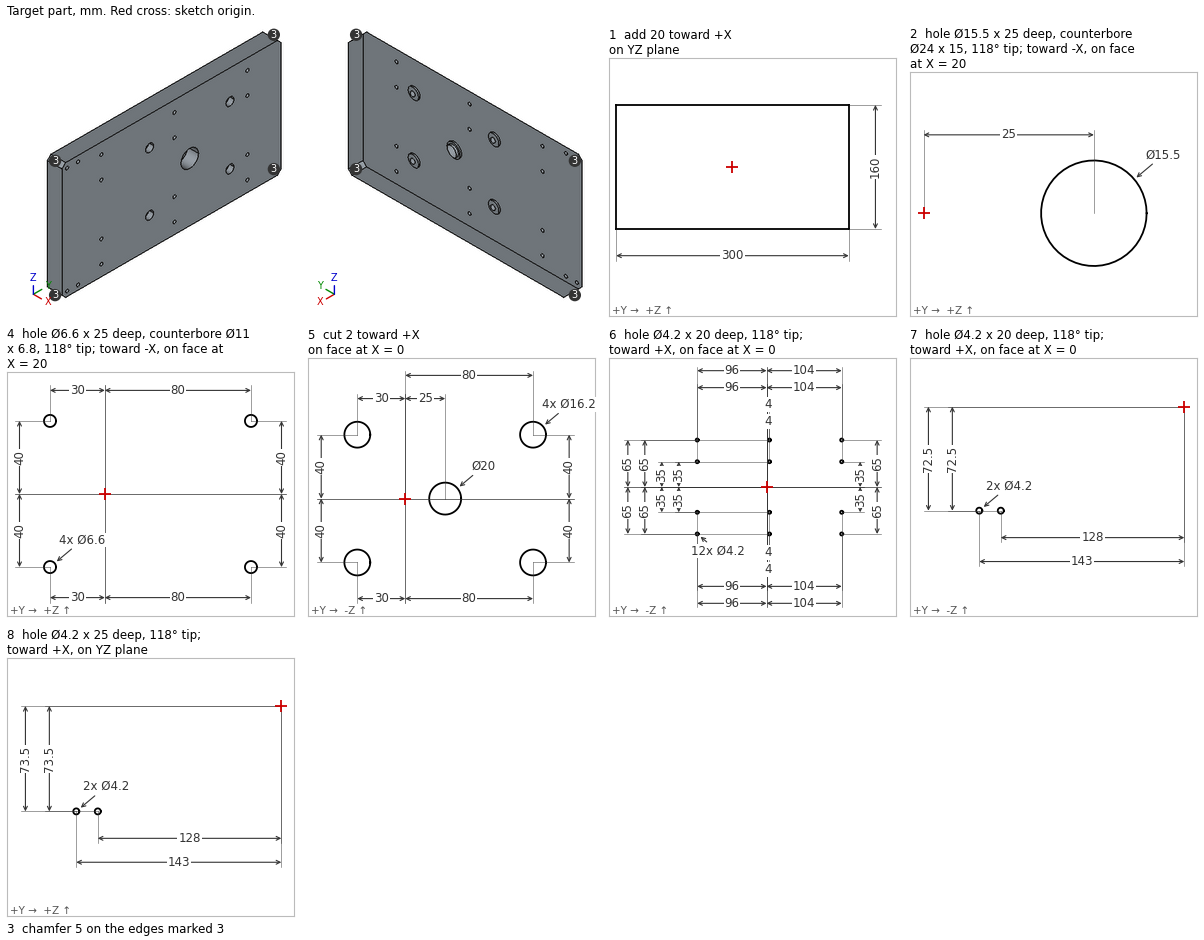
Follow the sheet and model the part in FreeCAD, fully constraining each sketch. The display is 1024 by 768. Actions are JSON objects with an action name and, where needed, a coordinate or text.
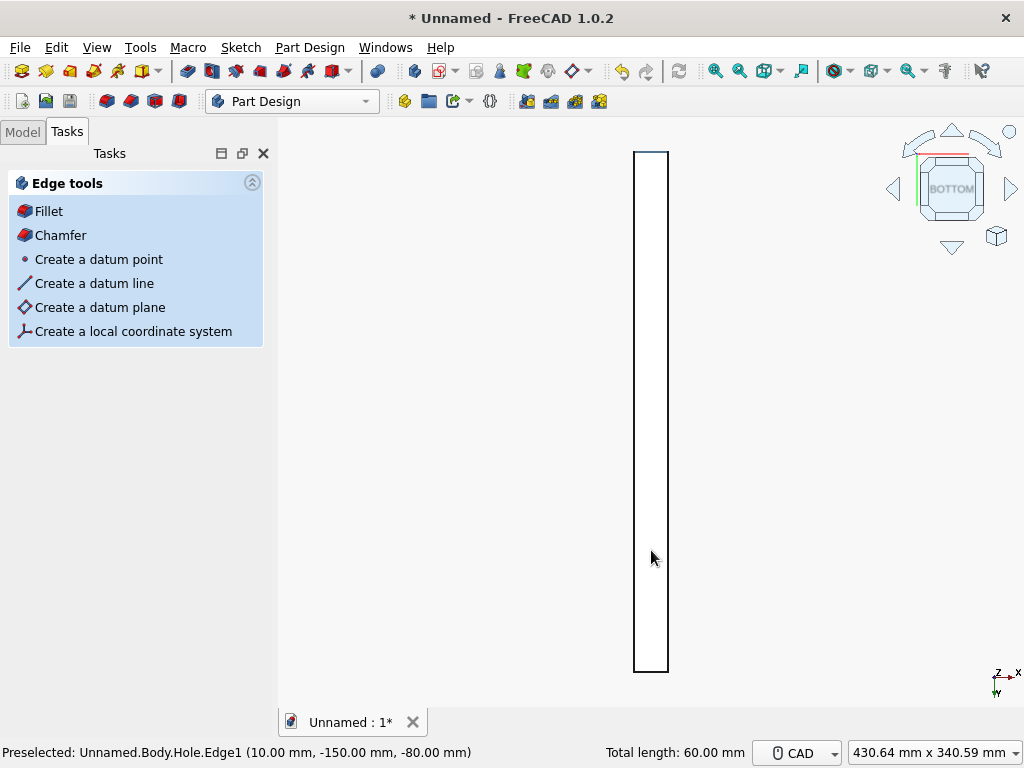
{"action": "left_click", "coordinate": [651, 671], "text": "ctrl"}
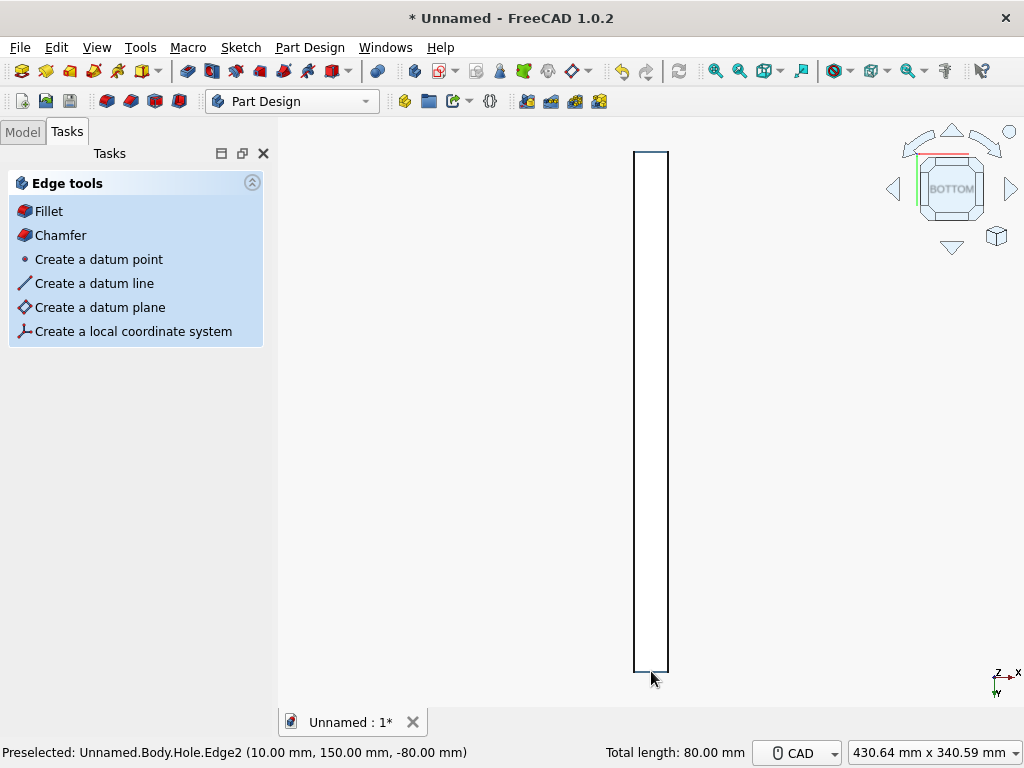
{"action": "left_click", "coordinate": [132, 102]}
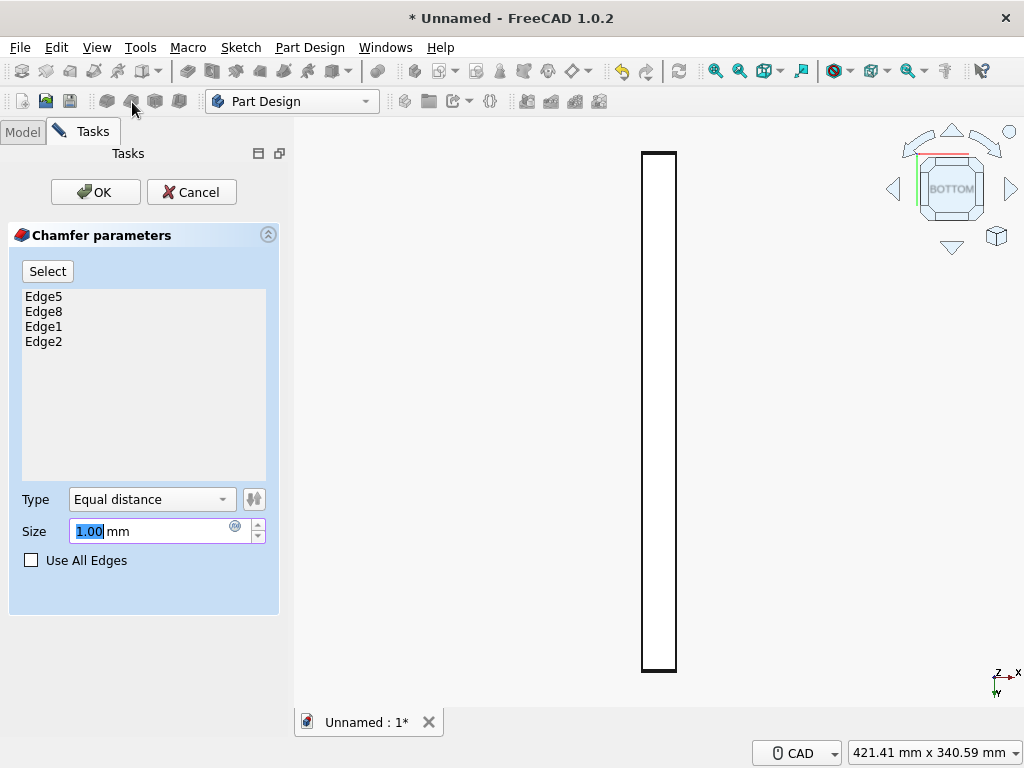
{"action": "type", "text": "5"}
{"action": "key", "text": "Tab"}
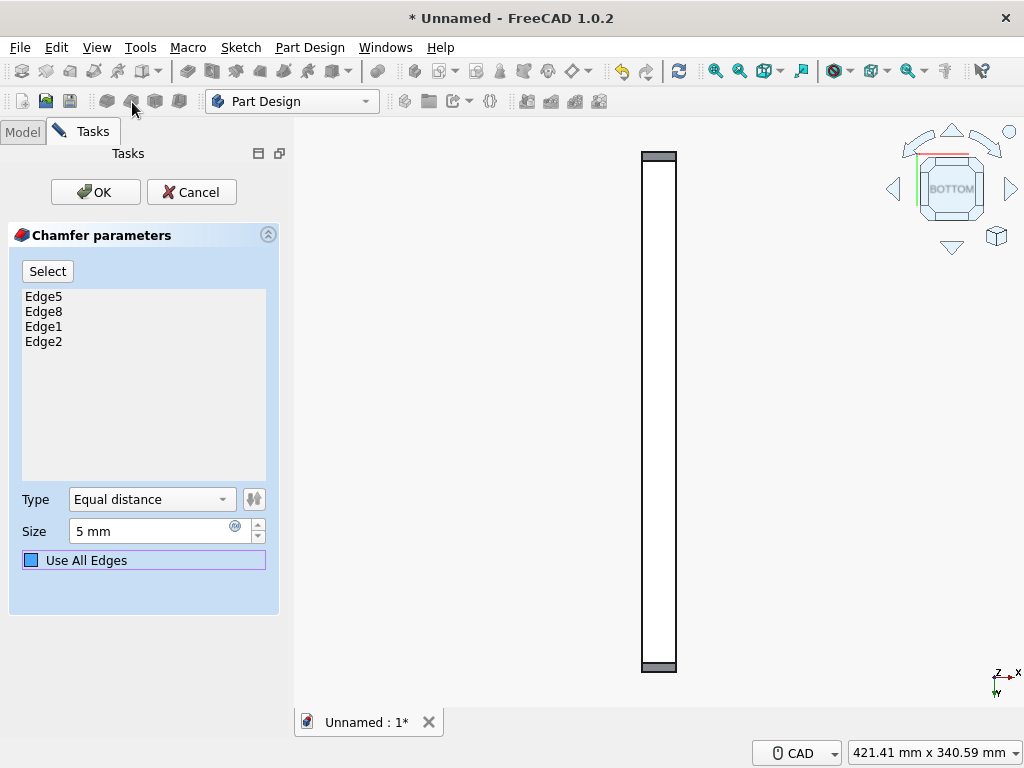
{"action": "left_click", "coordinate": [96, 192]}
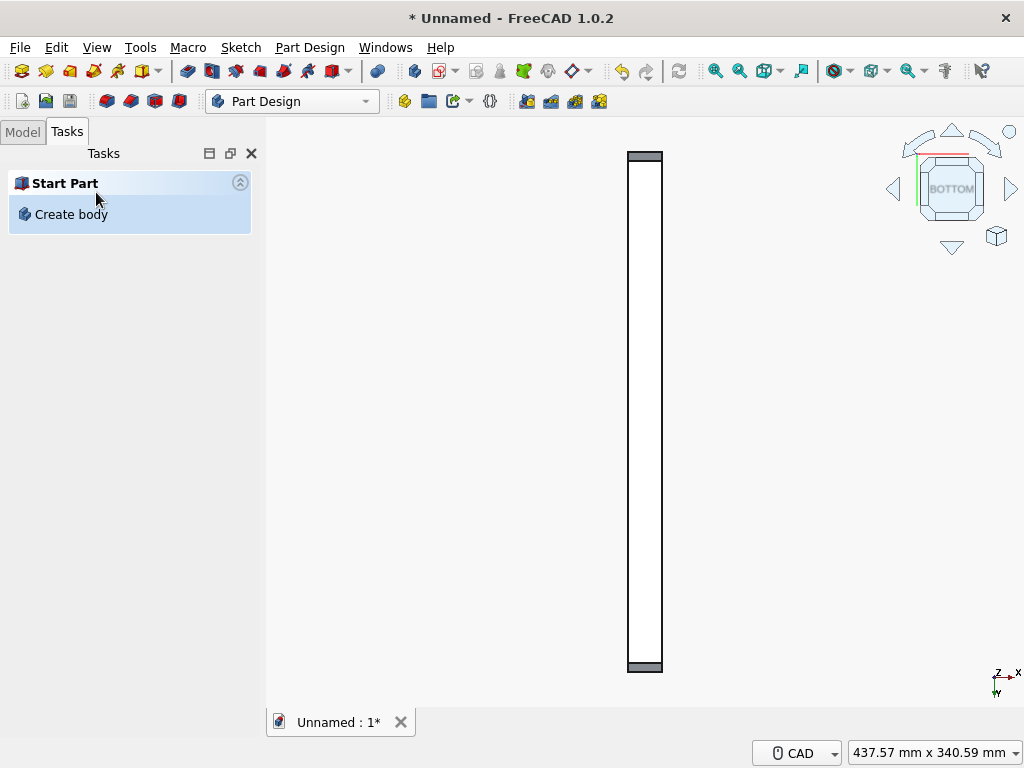
{"action": "key", "text": "0"}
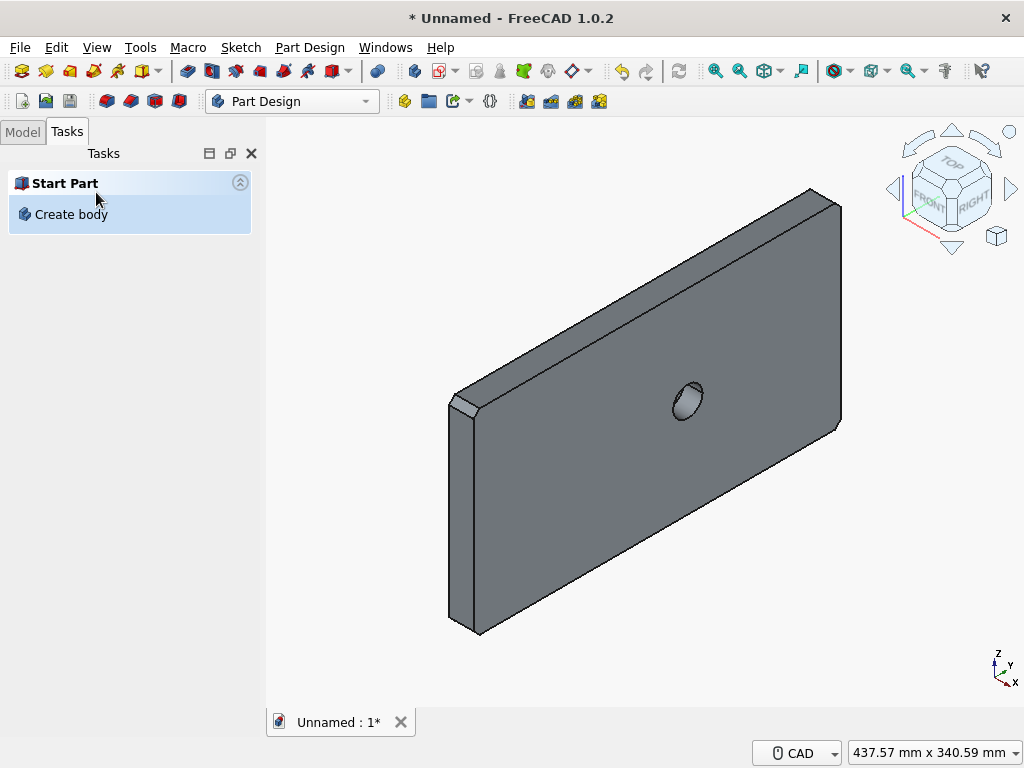
{"action": "left_click", "coordinate": [552, 479]}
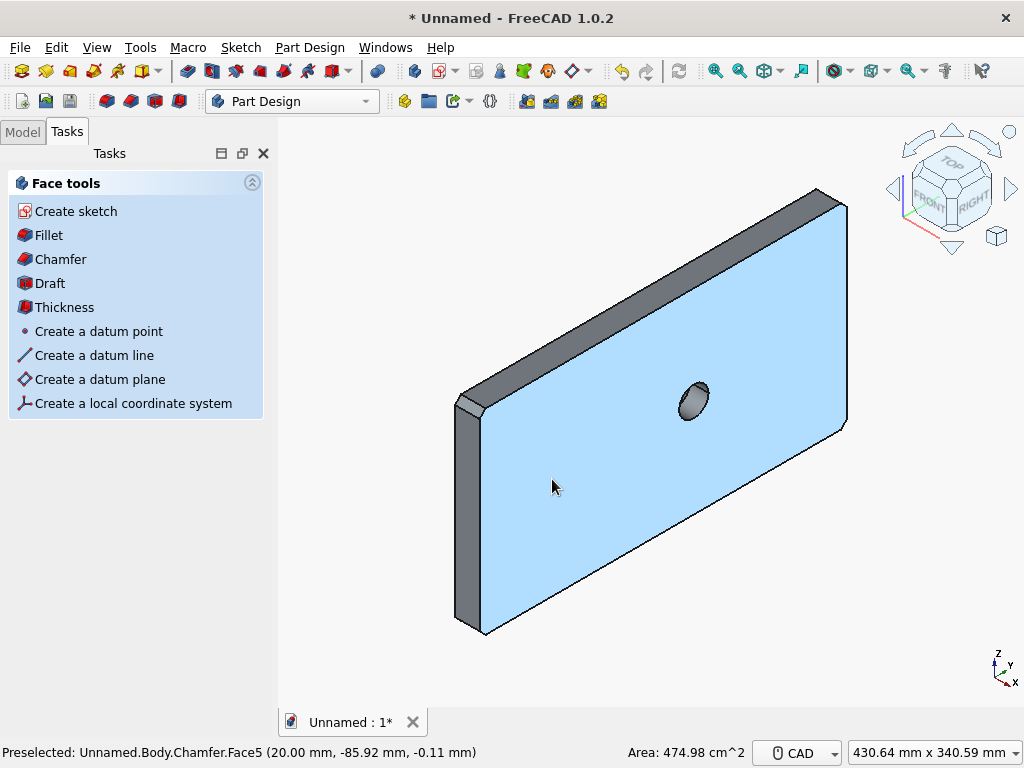
{"action": "left_click", "coordinate": [440, 72]}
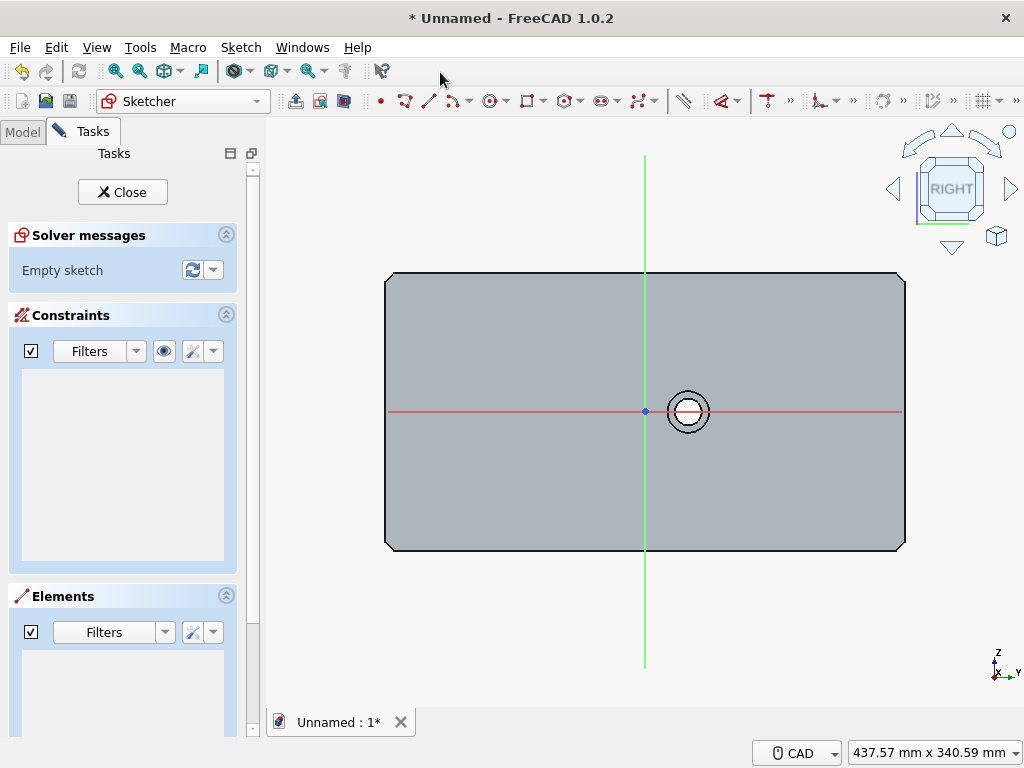
{"action": "scroll", "coordinate": [824, 412], "scroll_direction": "up", "scroll_amount": 3}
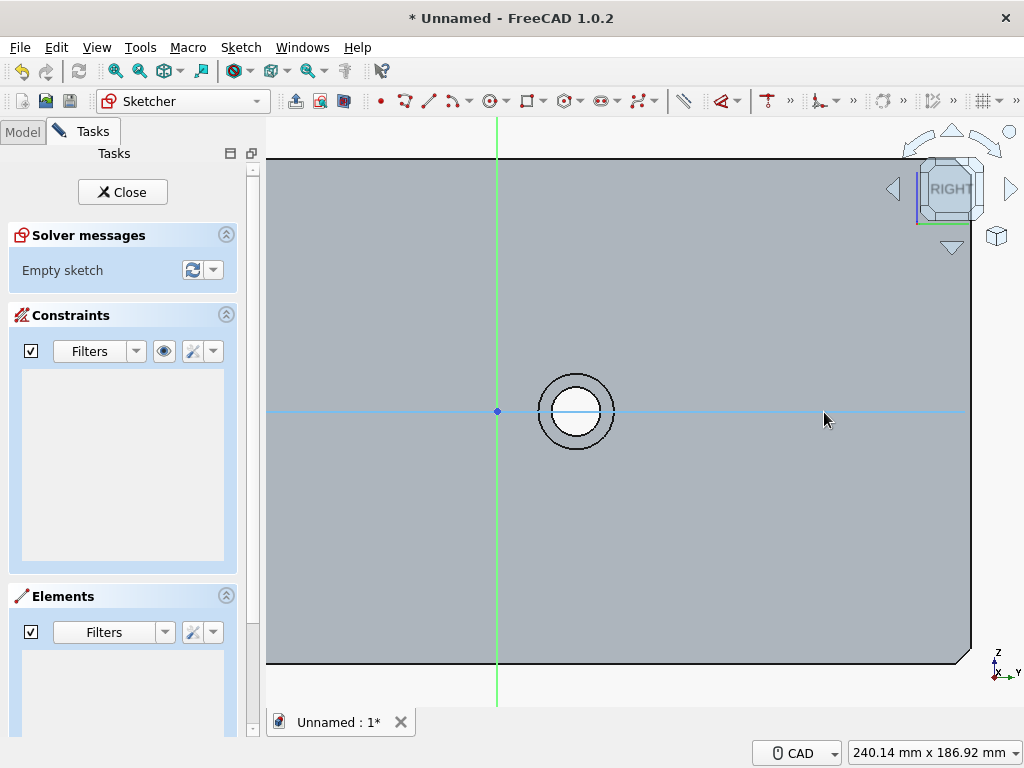
{"action": "left_click", "coordinate": [490, 102]}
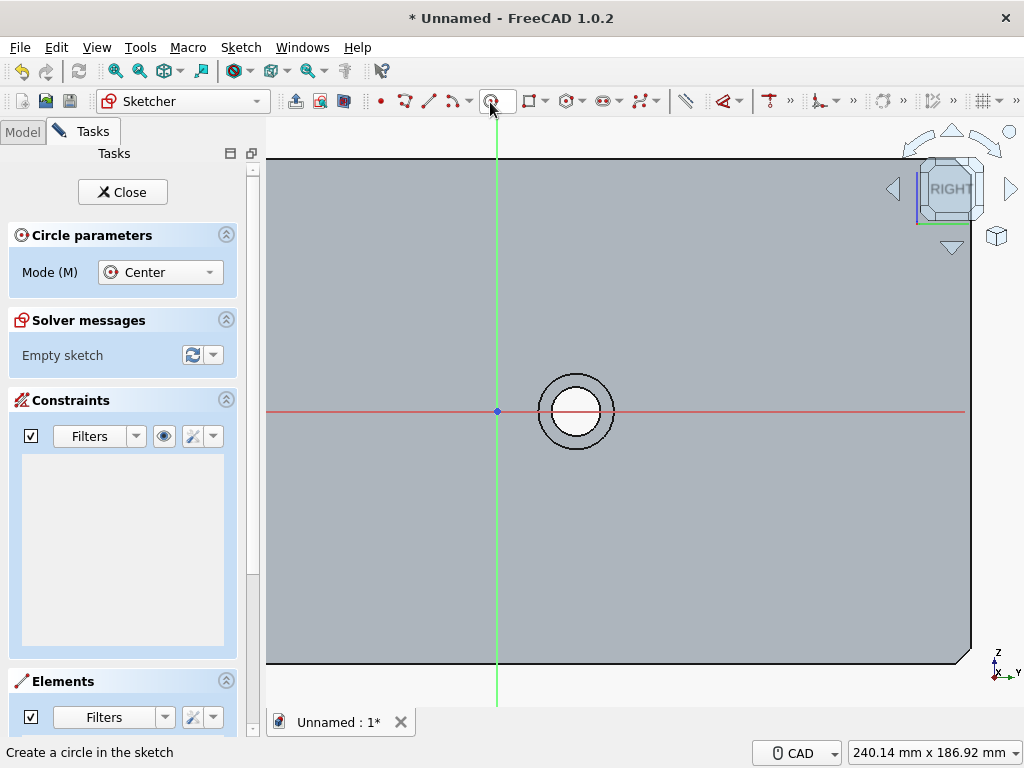
{"action": "scroll", "coordinate": [403, 538], "scroll_direction": "up", "scroll_amount": 4}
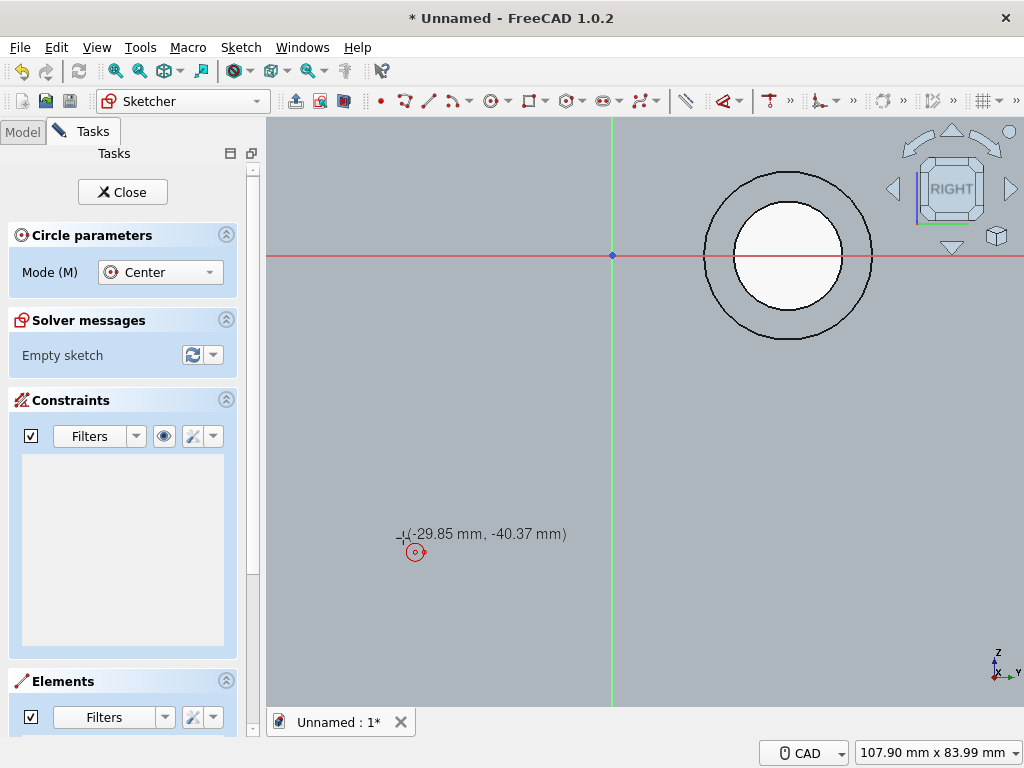
{"action": "left_click", "coordinate": [402, 537]}
{"action": "left_click", "coordinate": [418, 520]}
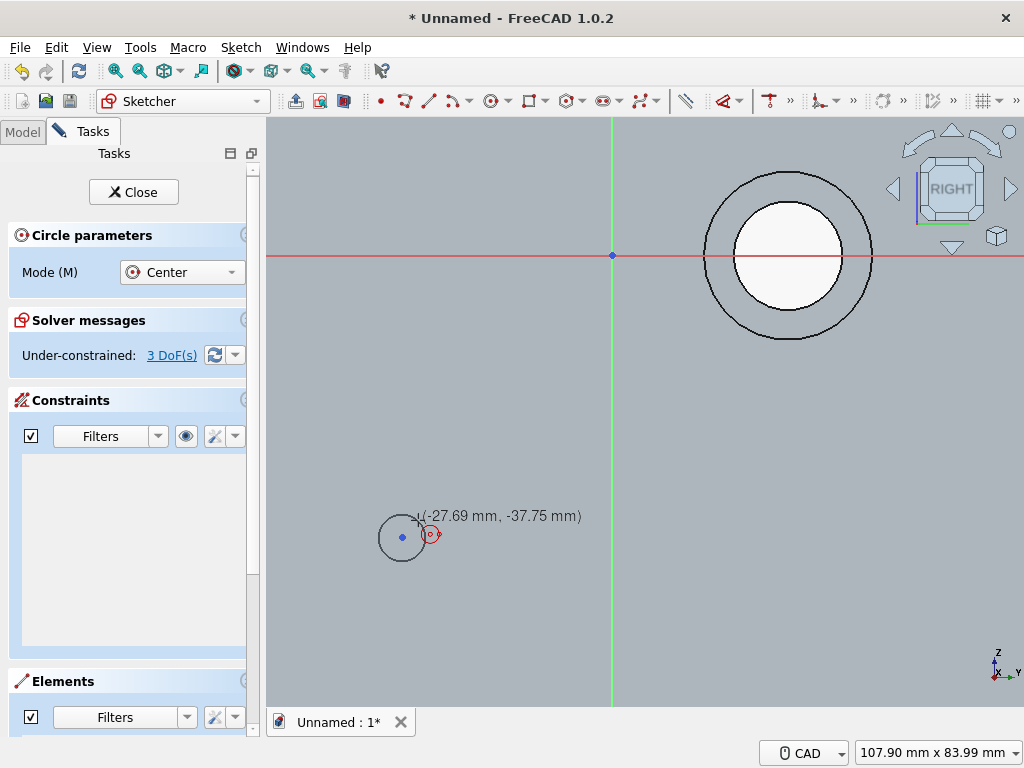
{"action": "scroll", "coordinate": [404, 539], "scroll_direction": "down", "scroll_amount": 4}